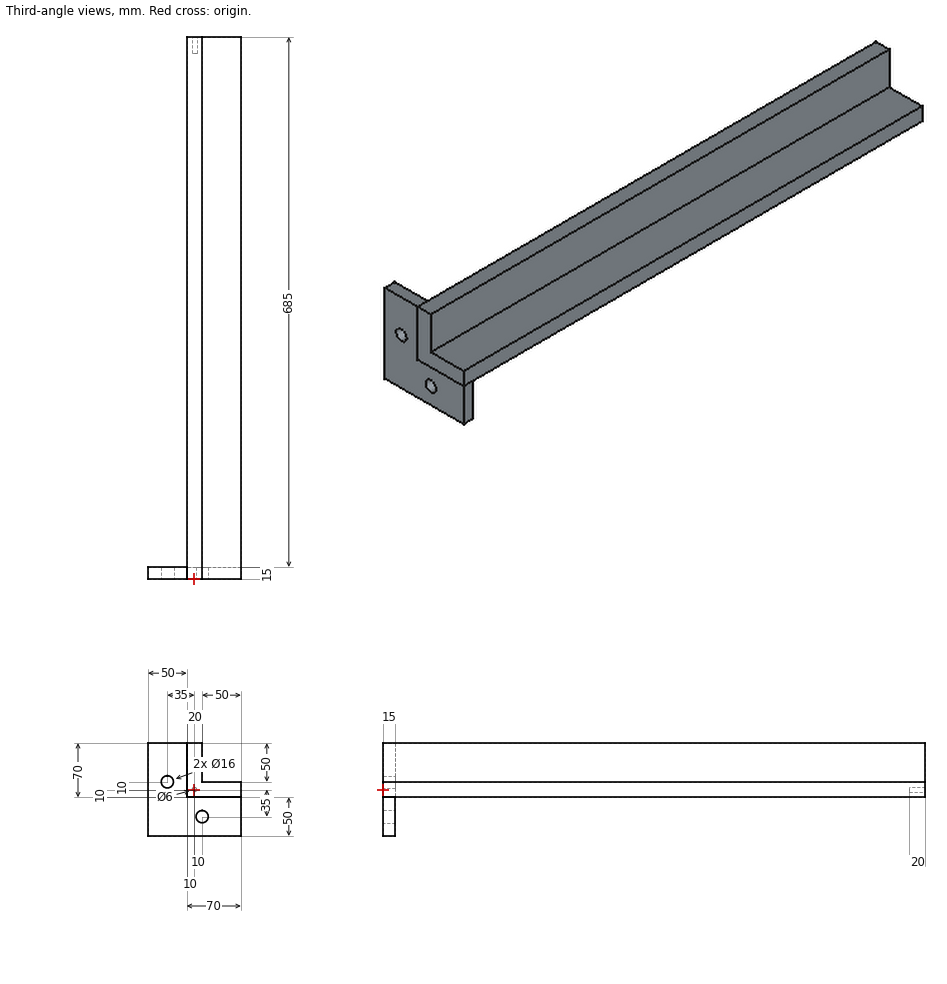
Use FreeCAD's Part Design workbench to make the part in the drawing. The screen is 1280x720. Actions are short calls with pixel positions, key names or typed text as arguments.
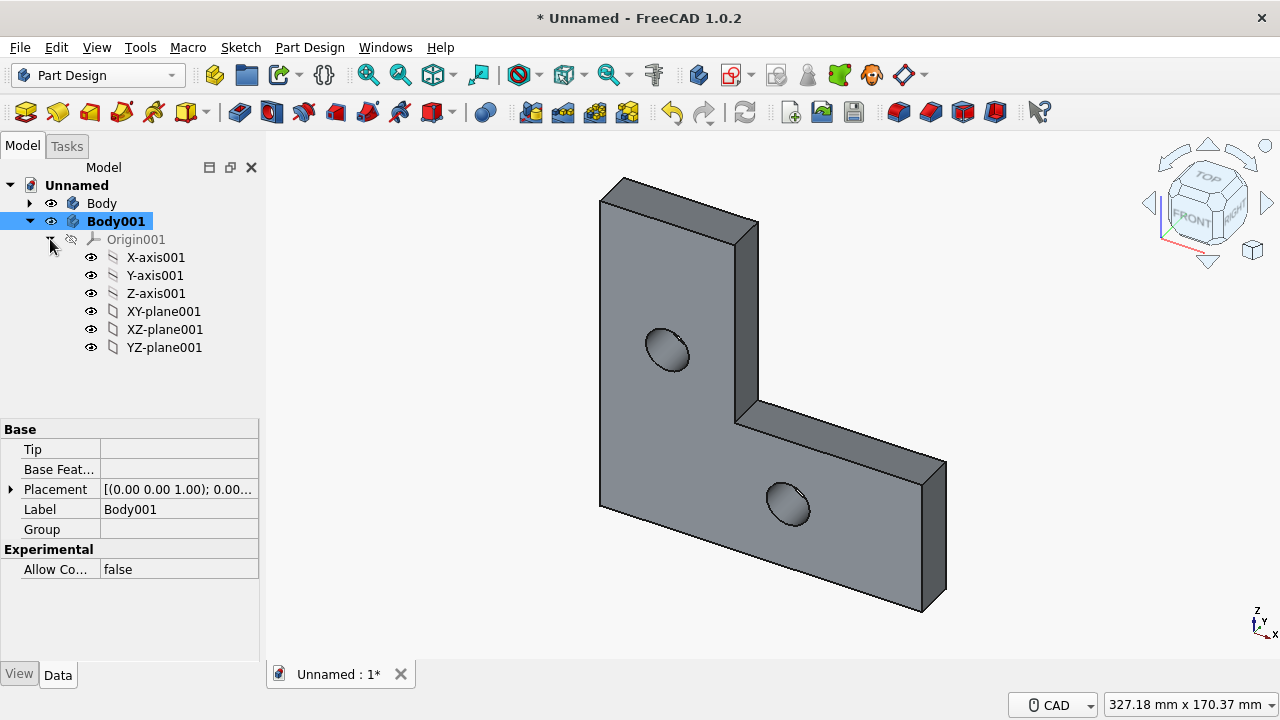
click(136, 329)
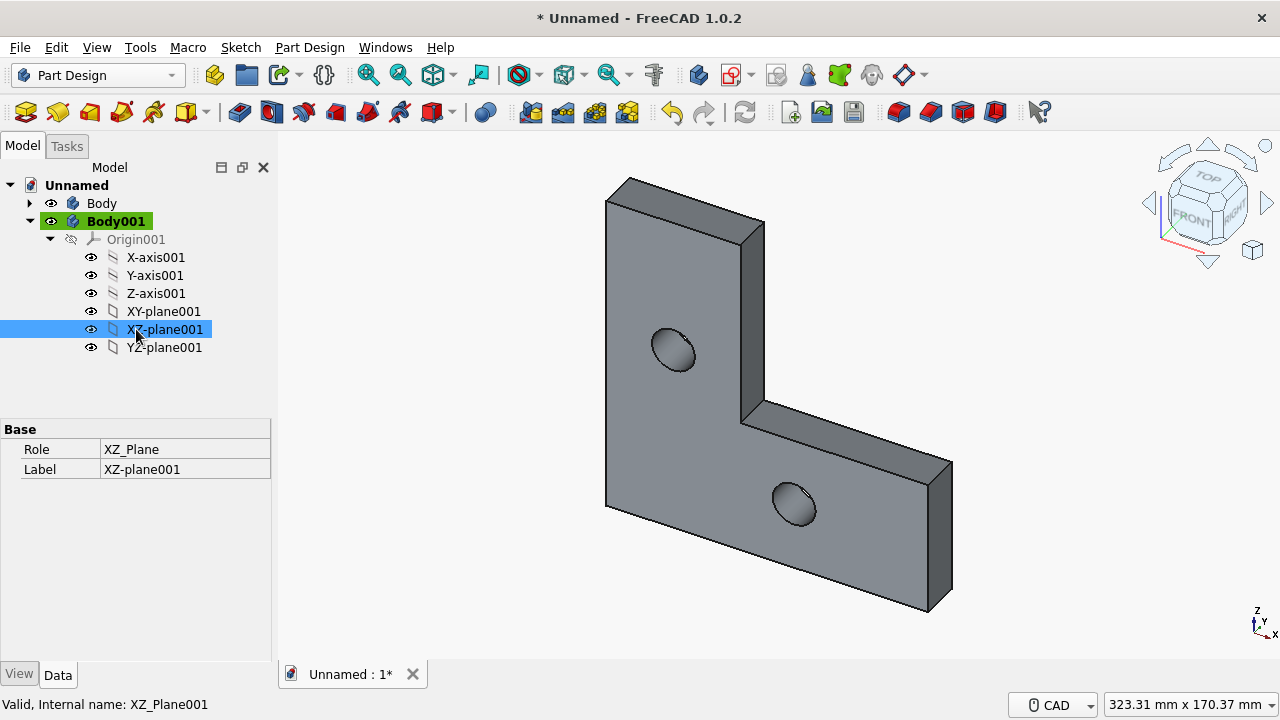
click(904, 76)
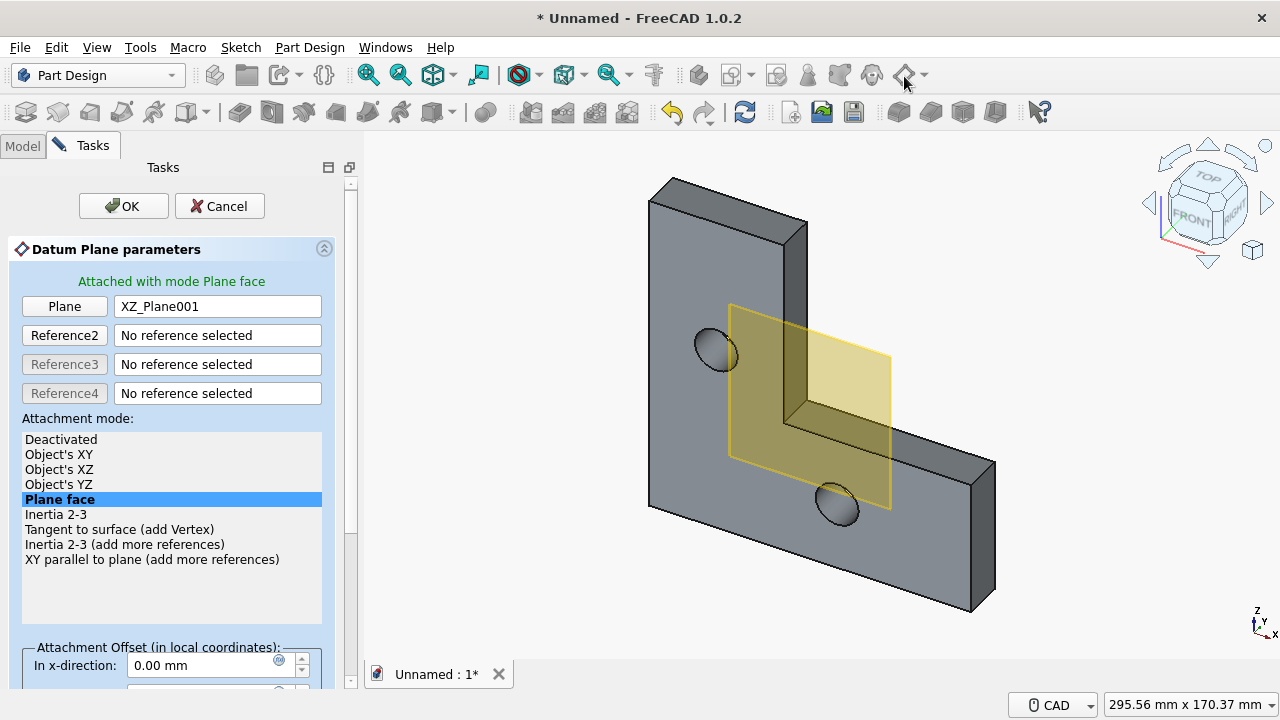
scroll(351, 432, down, 2)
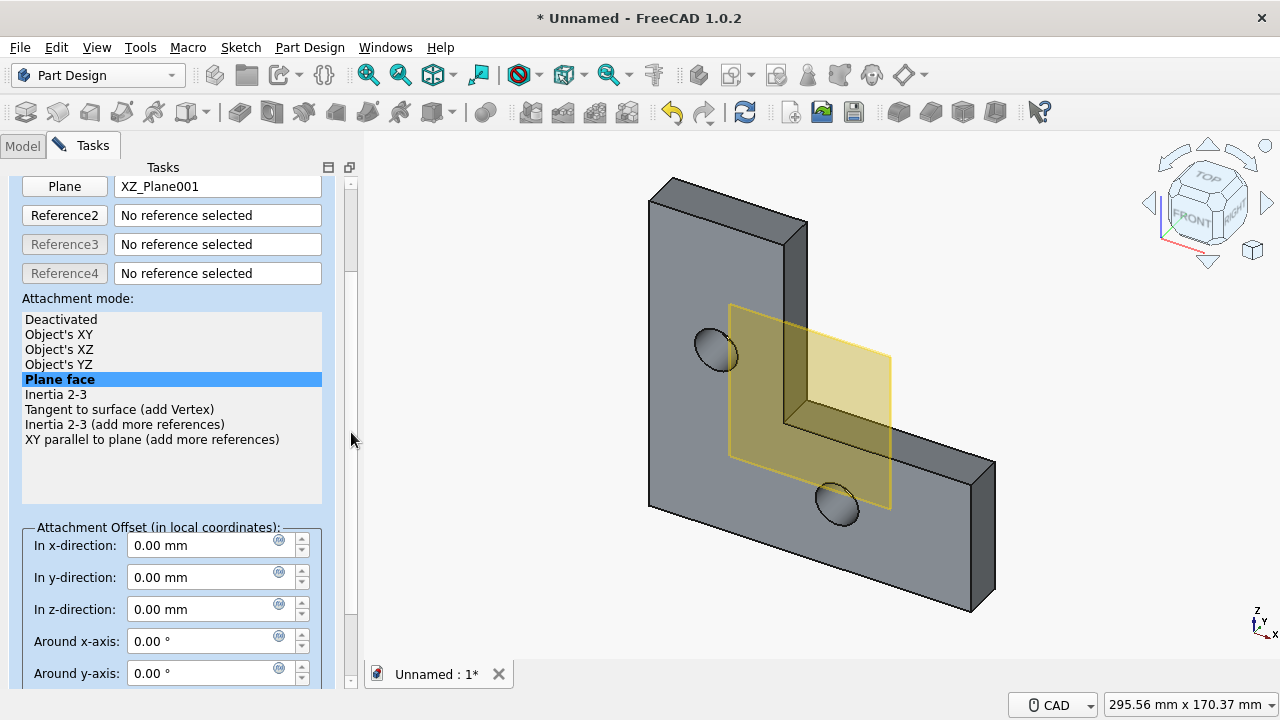
triple_click(210, 609)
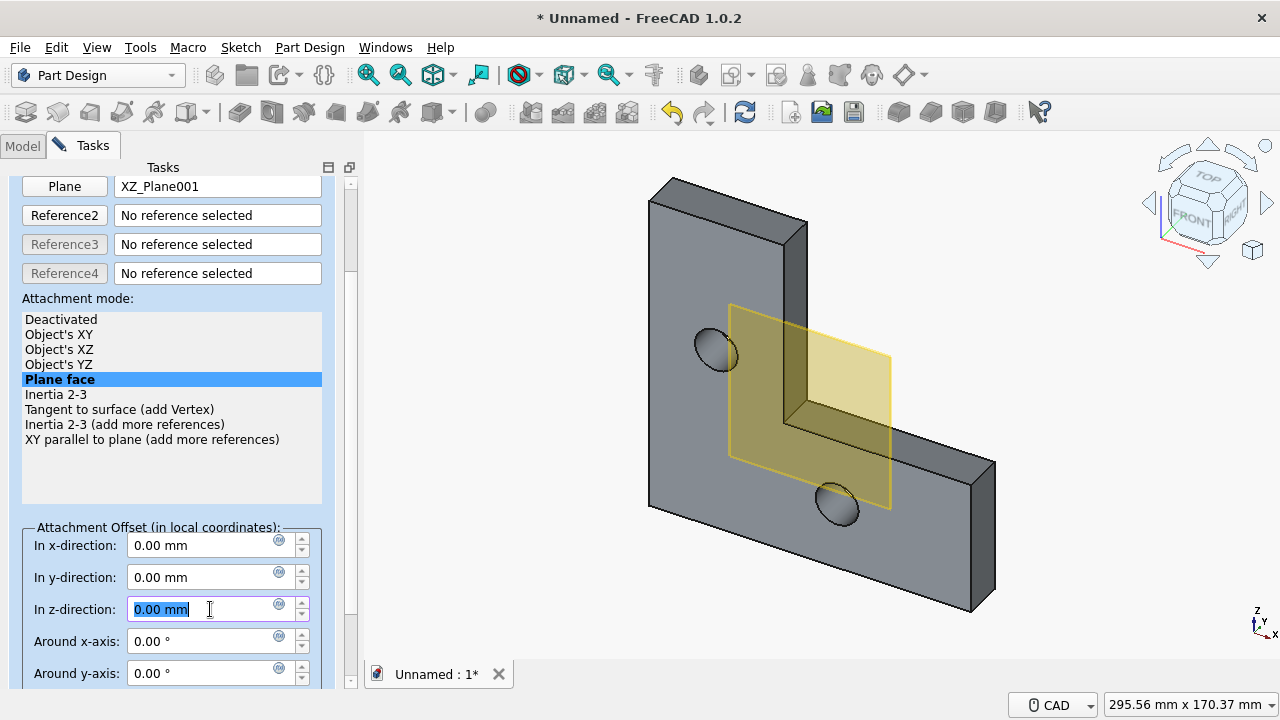
text(-15)
key(Tab)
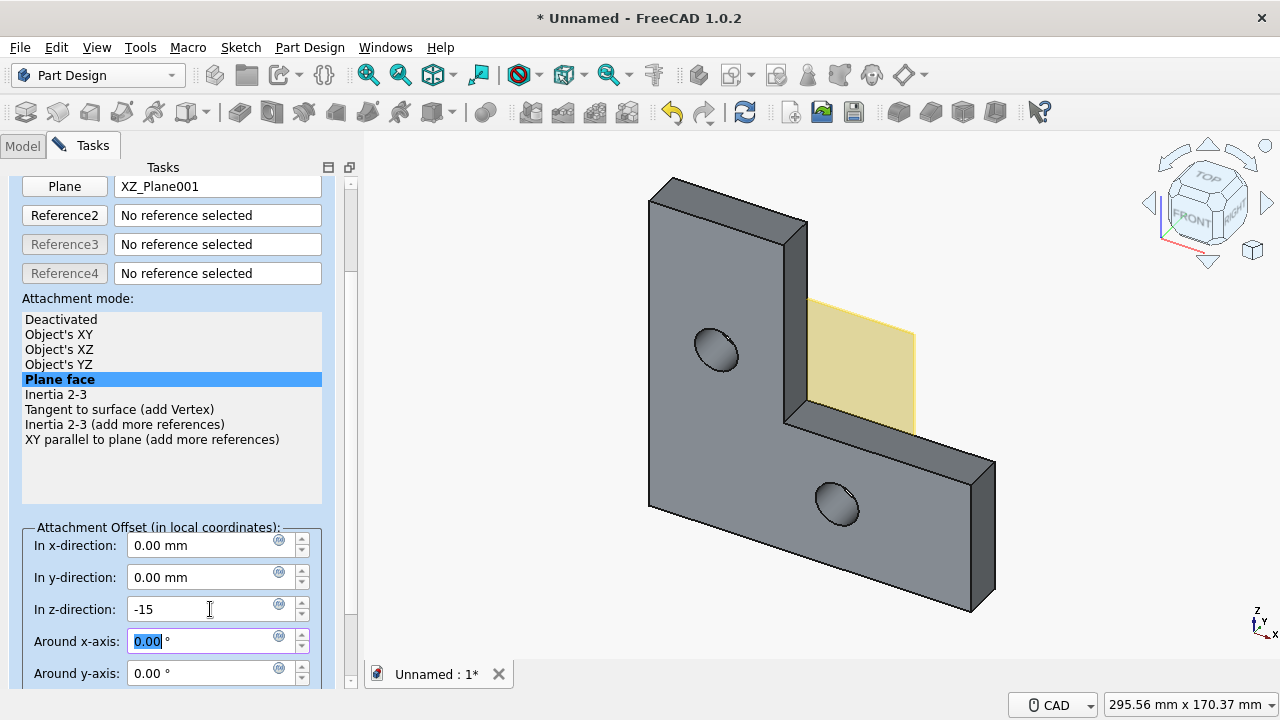
scroll(351, 432, up, 3)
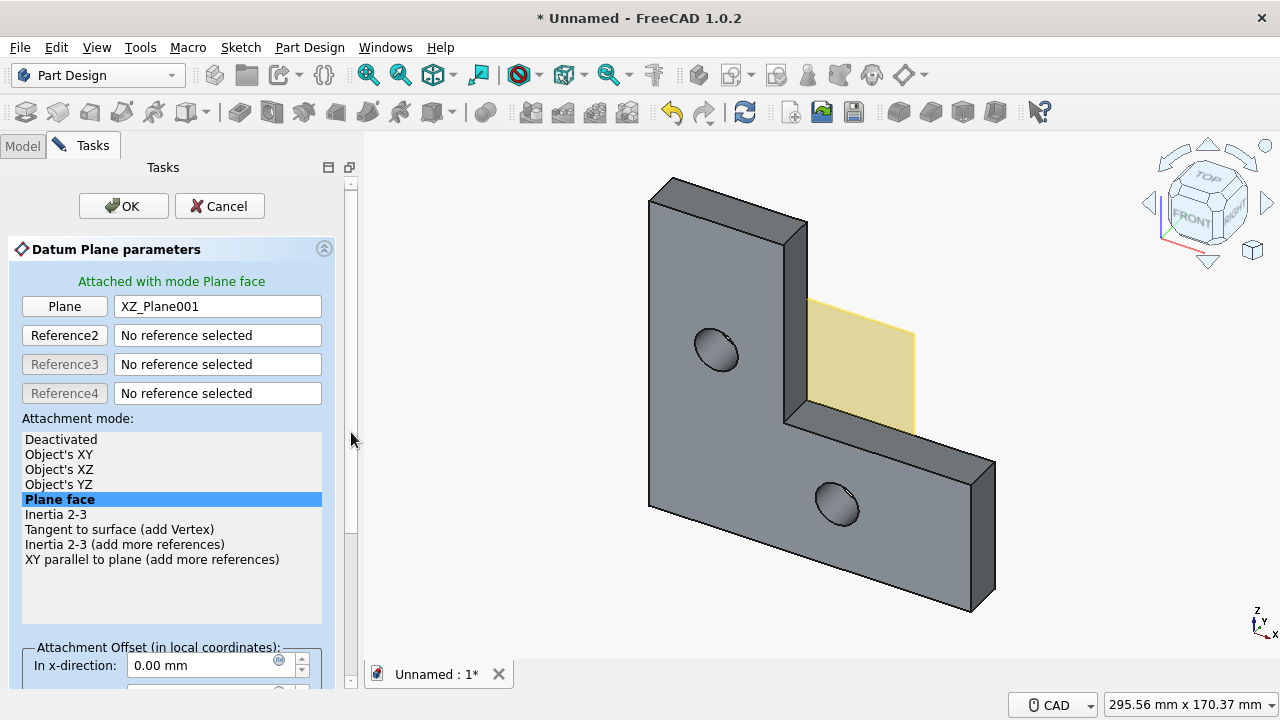
click(124, 206)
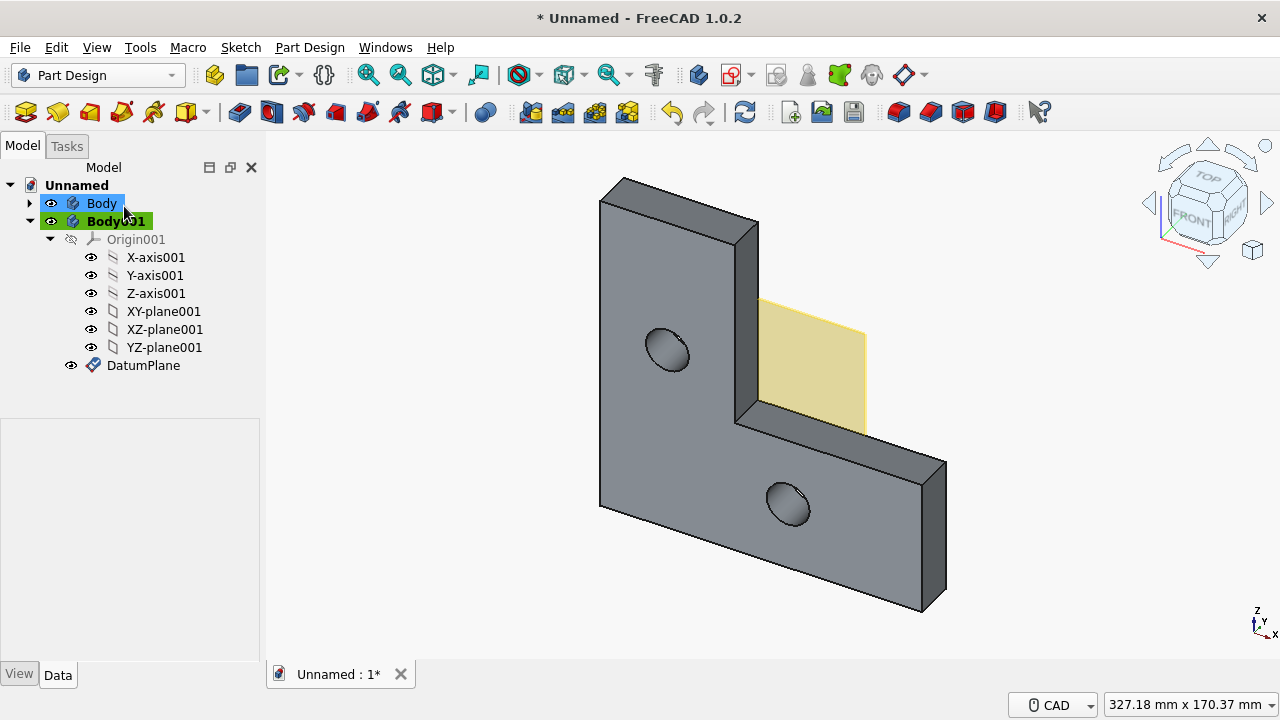
click(116, 365)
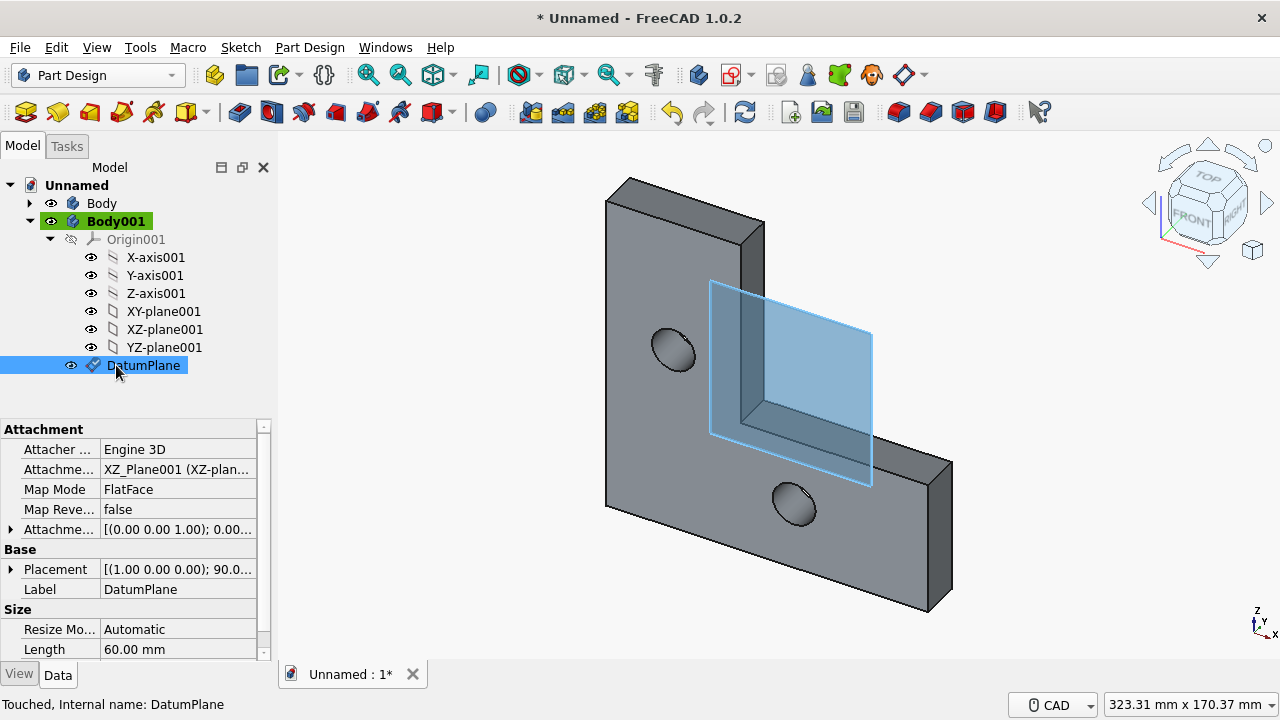
click(732, 76)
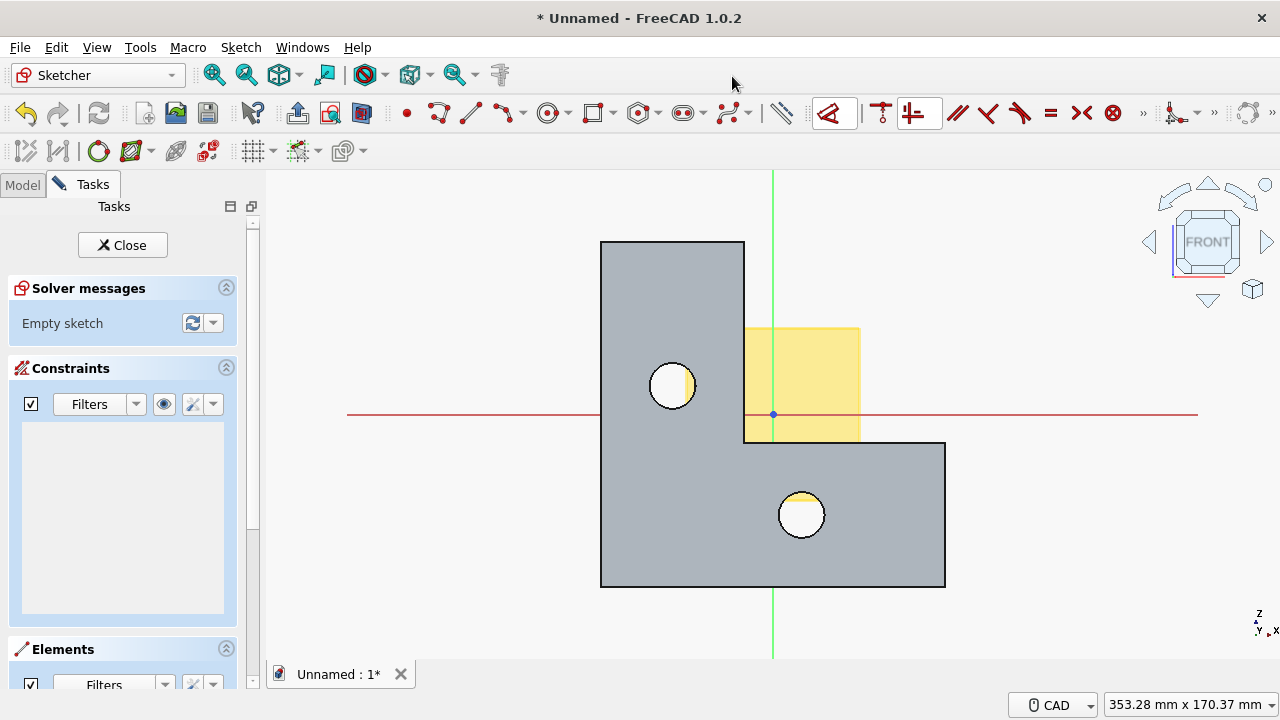
scroll(1115, 198, up, 2)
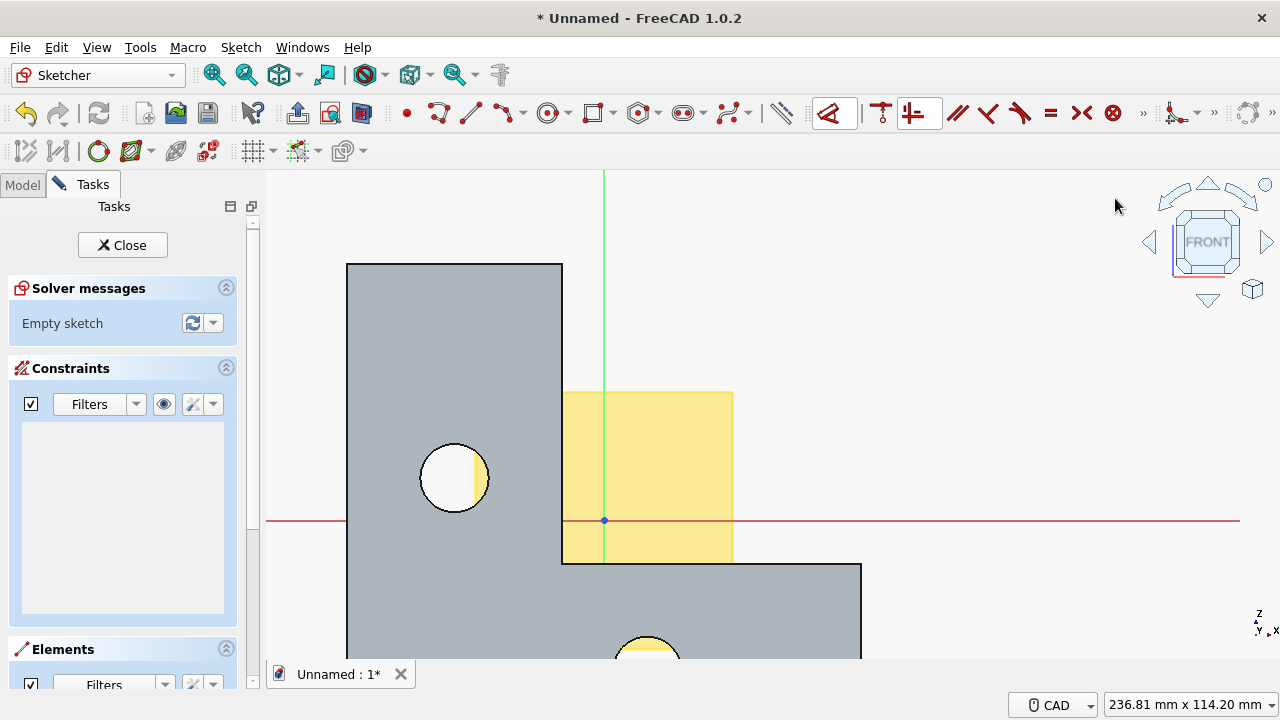
click(440, 114)